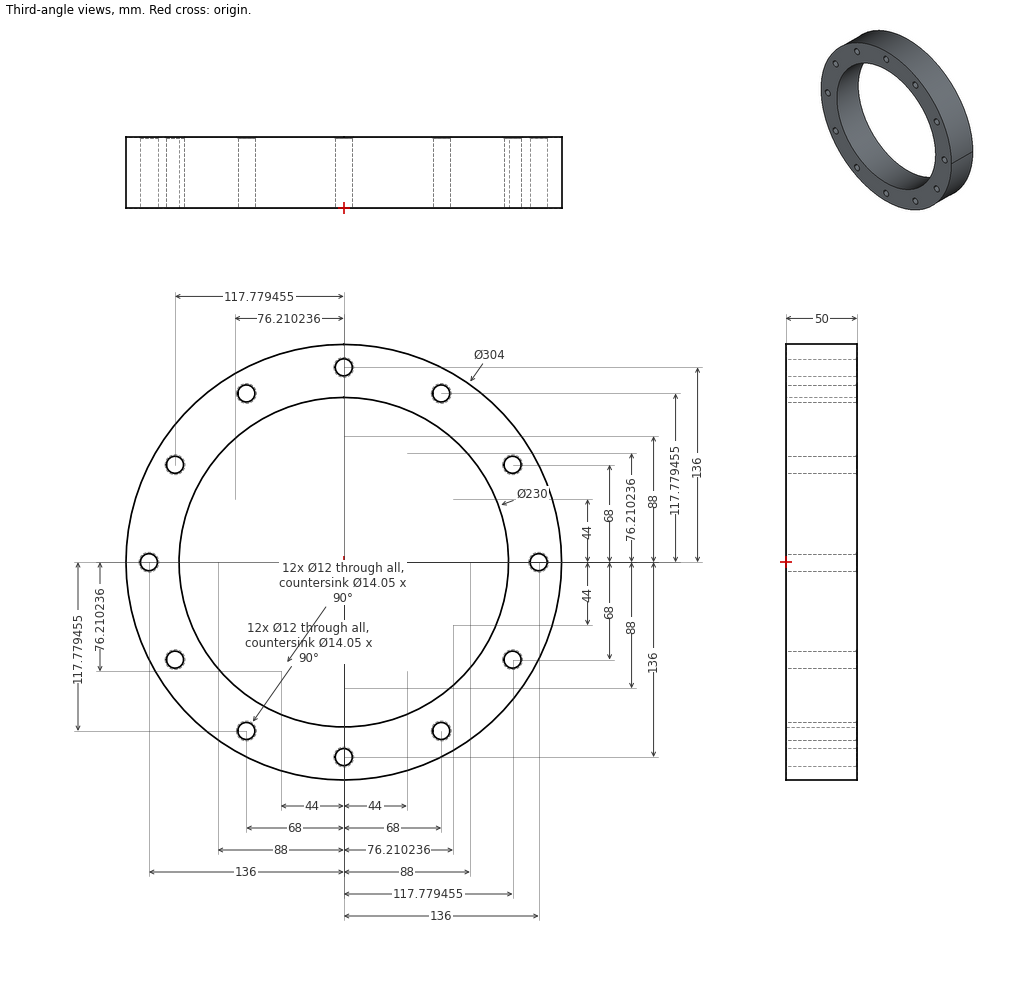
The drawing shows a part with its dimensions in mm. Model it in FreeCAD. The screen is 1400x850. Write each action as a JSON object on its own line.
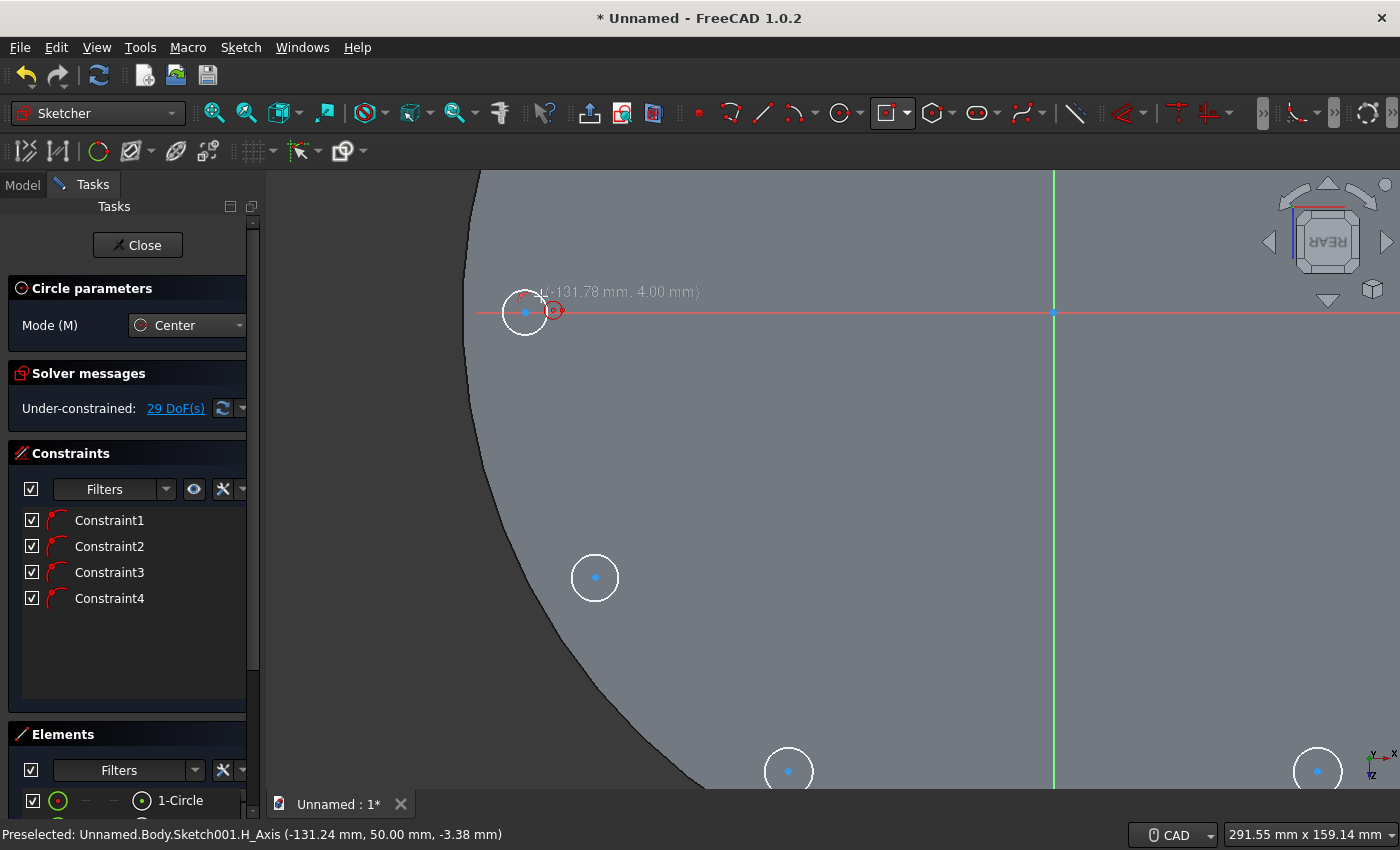
{"action": "scroll", "coordinate": [596, 577], "scroll_direction": "down", "scroll_amount": 5}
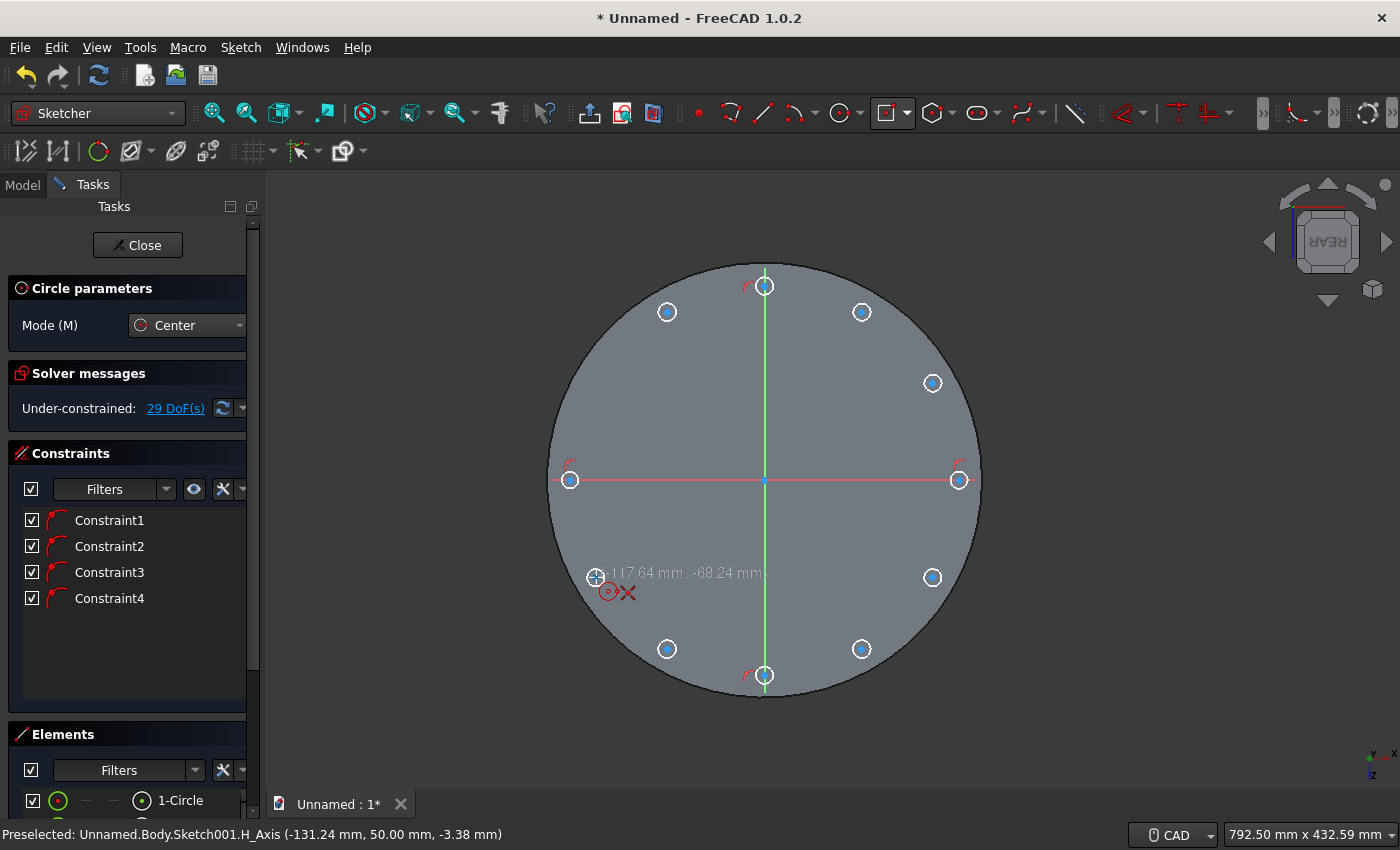
{"action": "scroll", "coordinate": [596, 383], "scroll_direction": "up", "scroll_amount": 5}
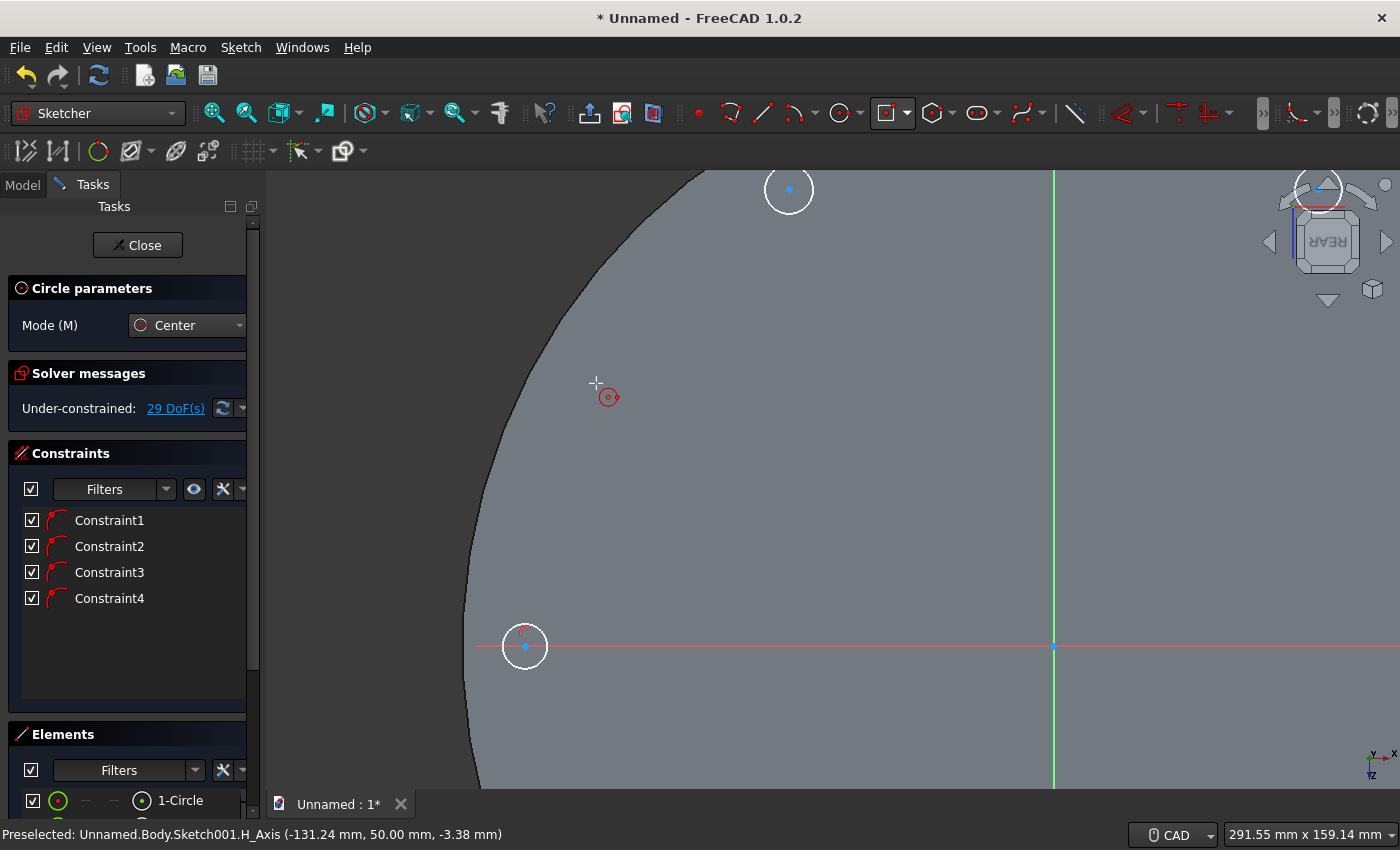
{"action": "left_click", "coordinate": [595, 382]}
{"action": "left_click", "coordinate": [612, 365]}
{"action": "key", "text": "Escape"}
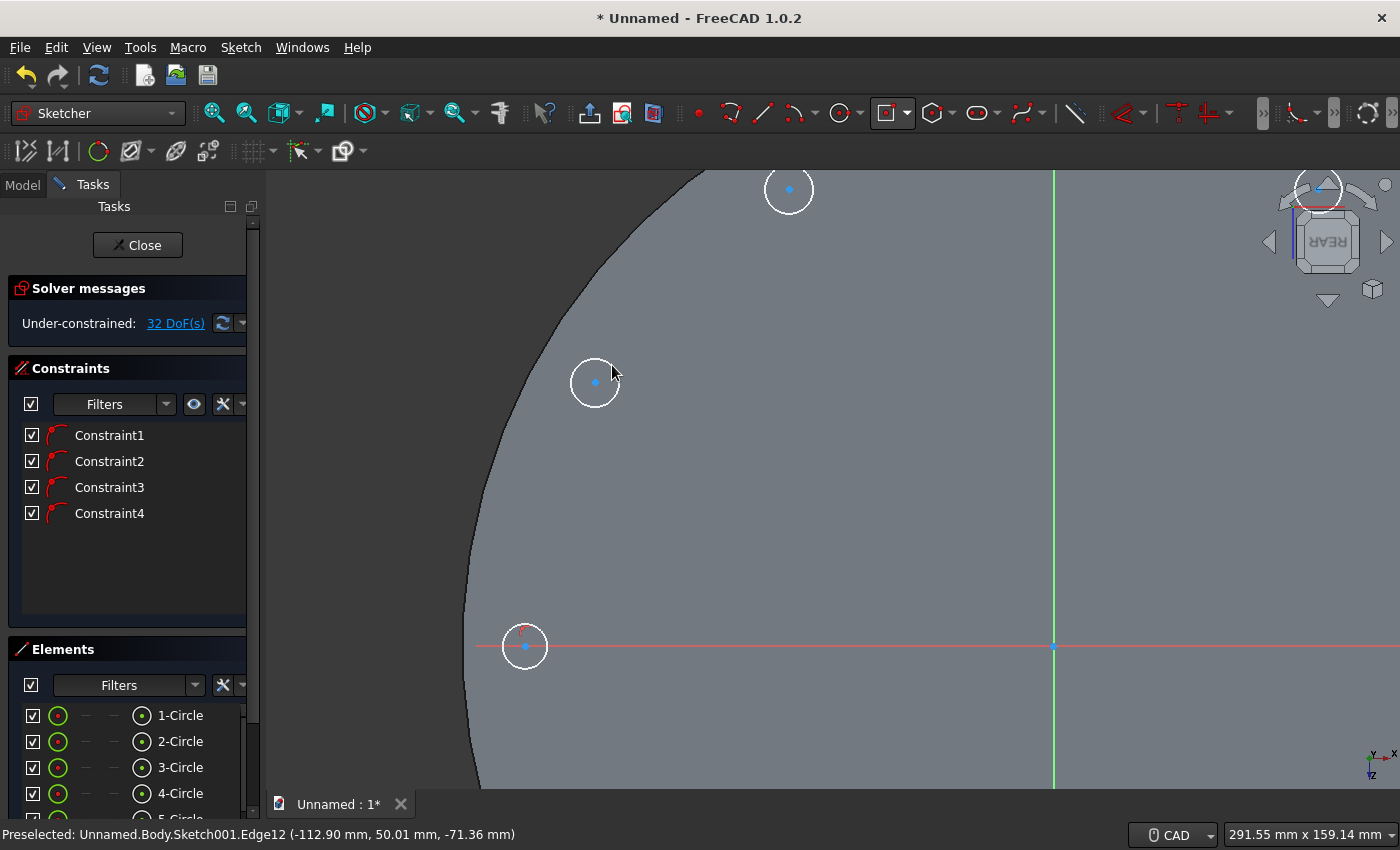
{"action": "left_click", "coordinate": [772, 207]}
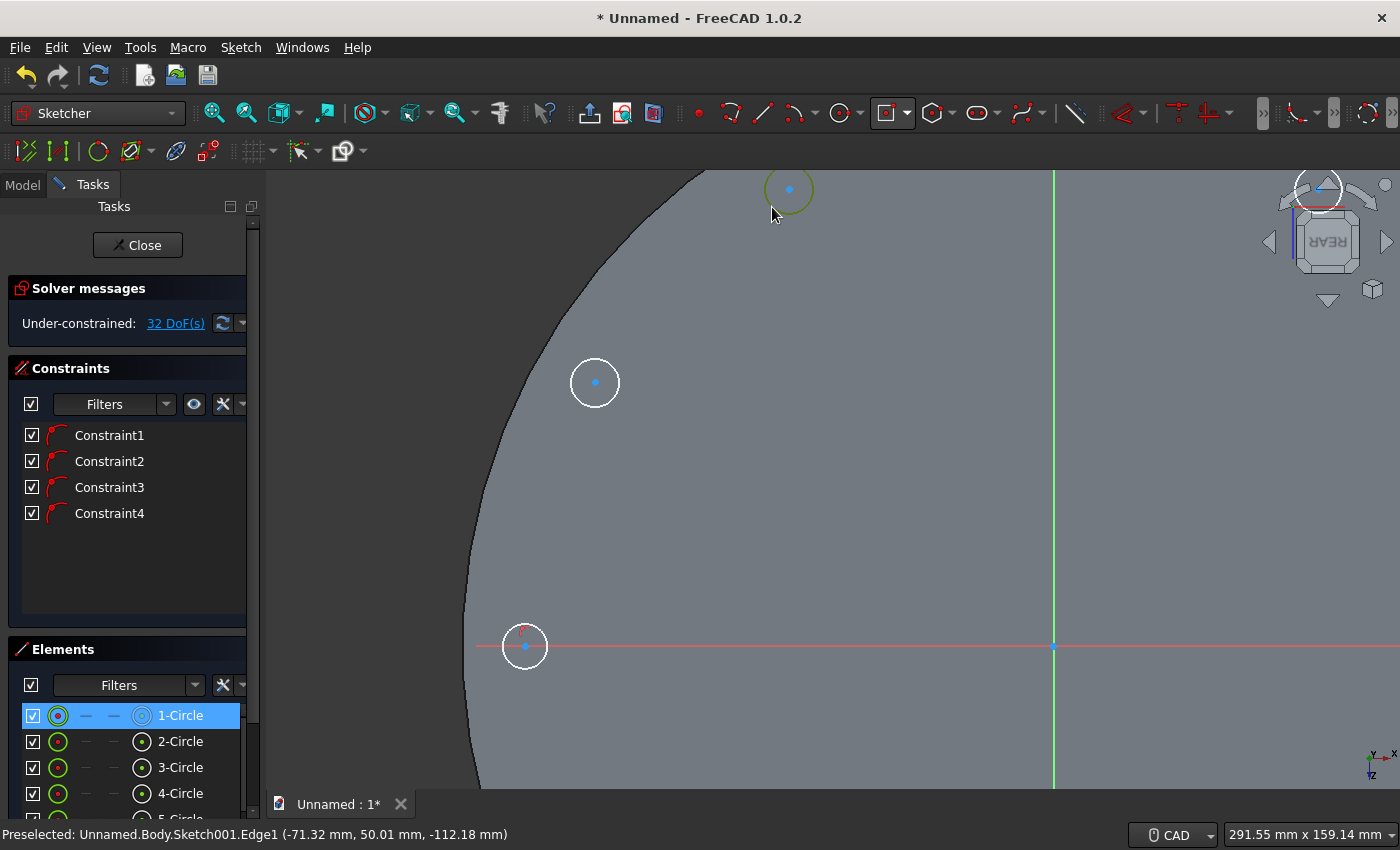
{"action": "scroll", "coordinate": [596, 382], "scroll_direction": "down", "scroll_amount": 5}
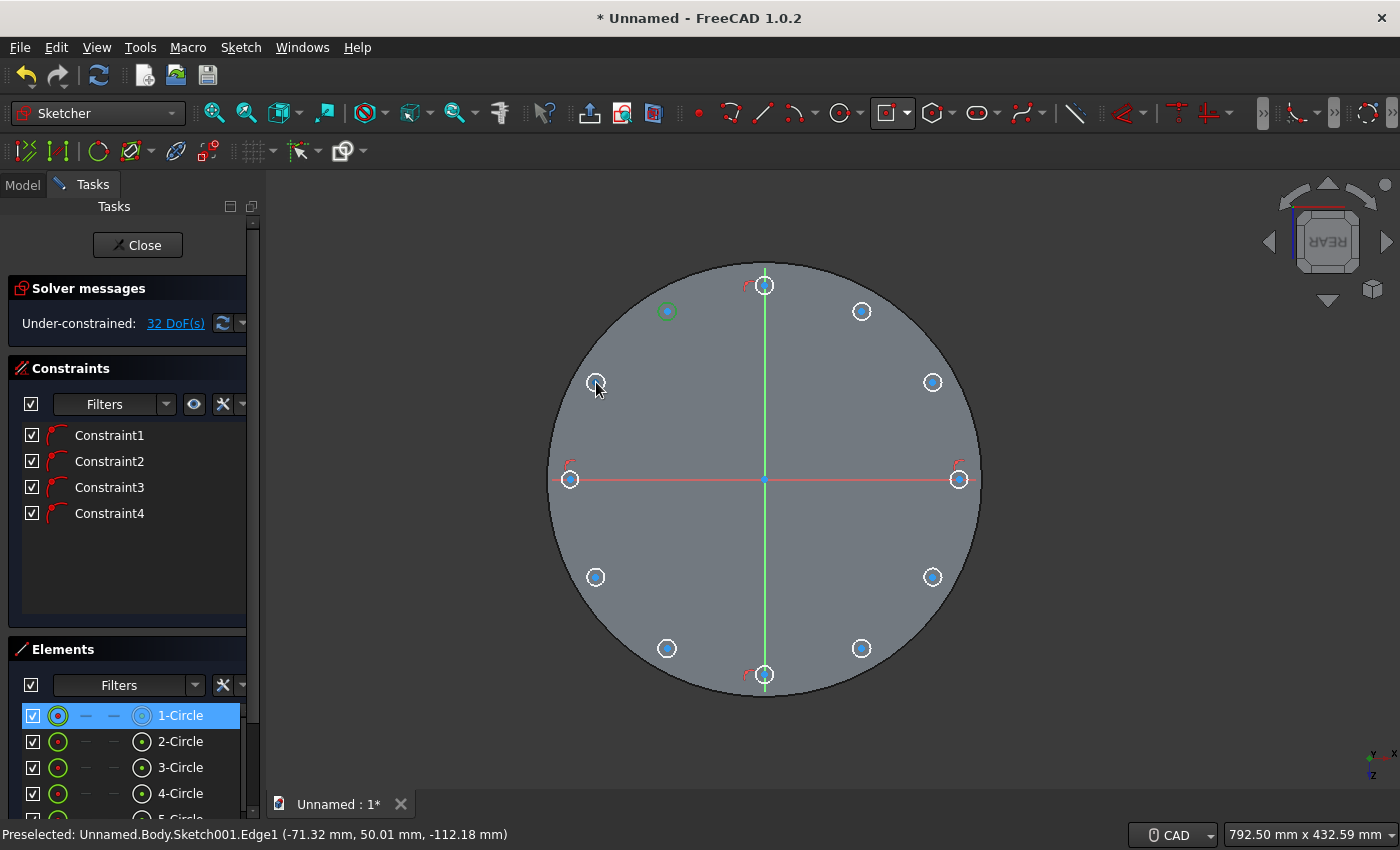
{"action": "scroll", "coordinate": [771, 279], "scroll_direction": "up", "scroll_amount": 5}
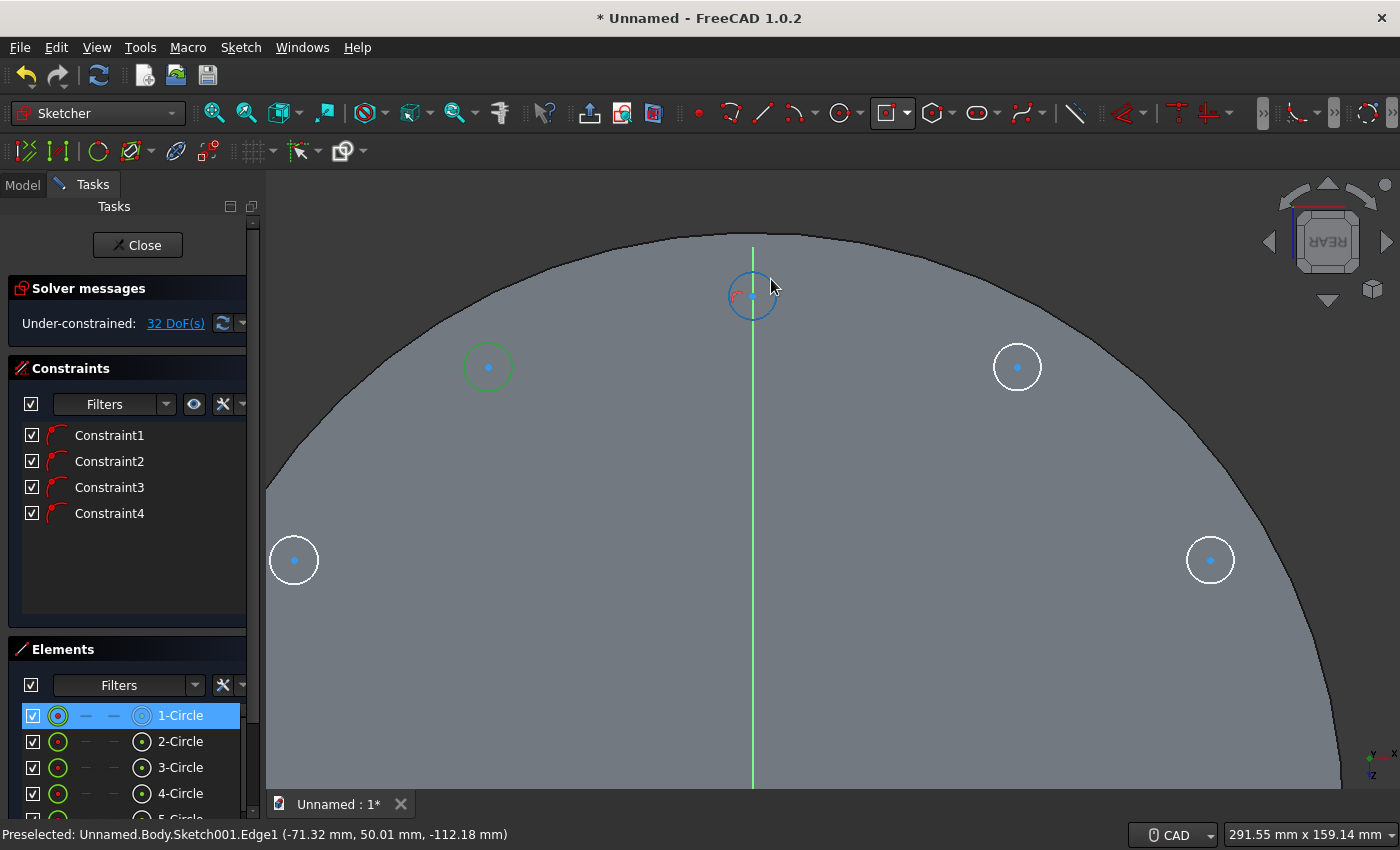
{"action": "left_click", "coordinate": [769, 279]}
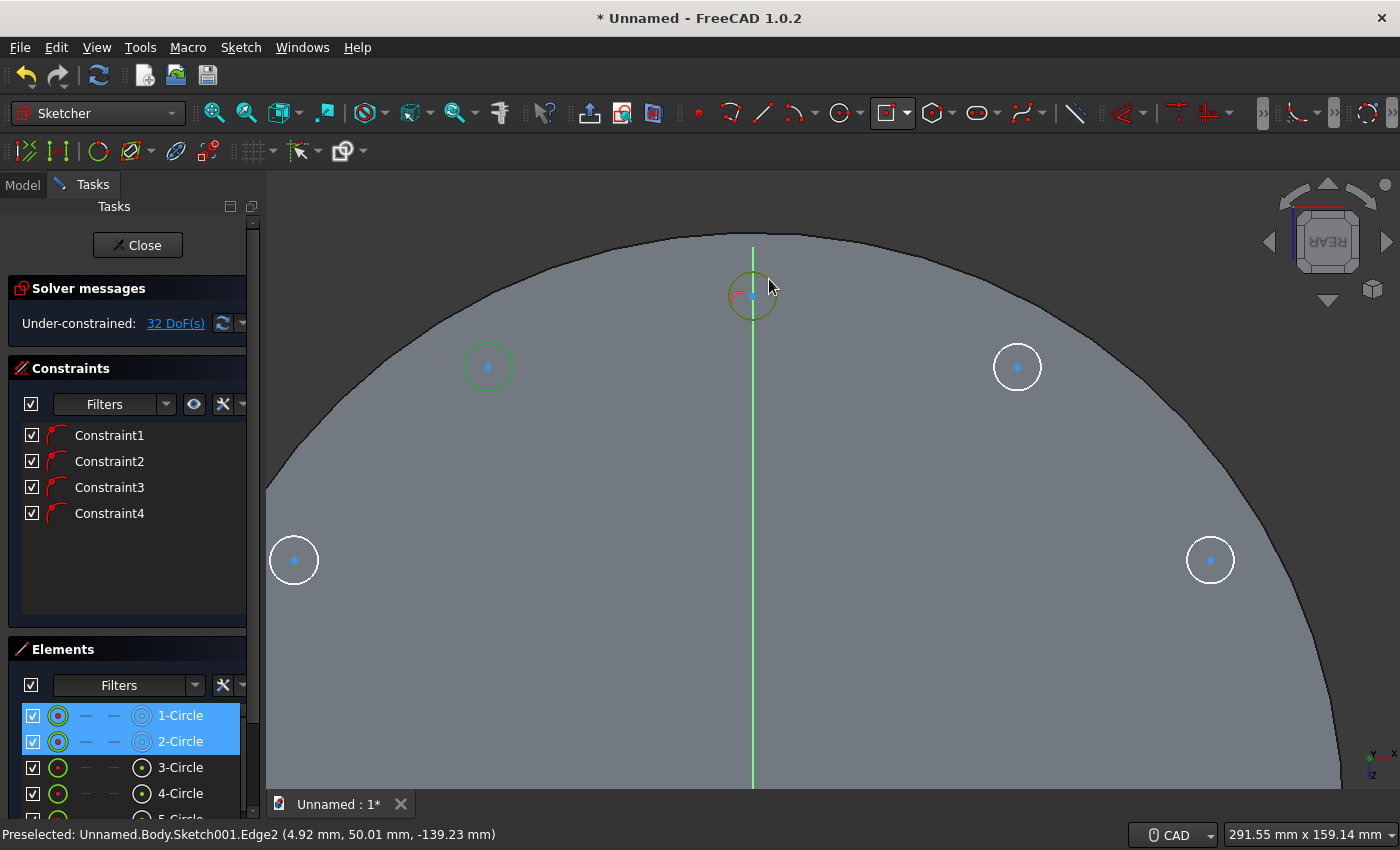
{"action": "left_click", "coordinate": [1034, 351]}